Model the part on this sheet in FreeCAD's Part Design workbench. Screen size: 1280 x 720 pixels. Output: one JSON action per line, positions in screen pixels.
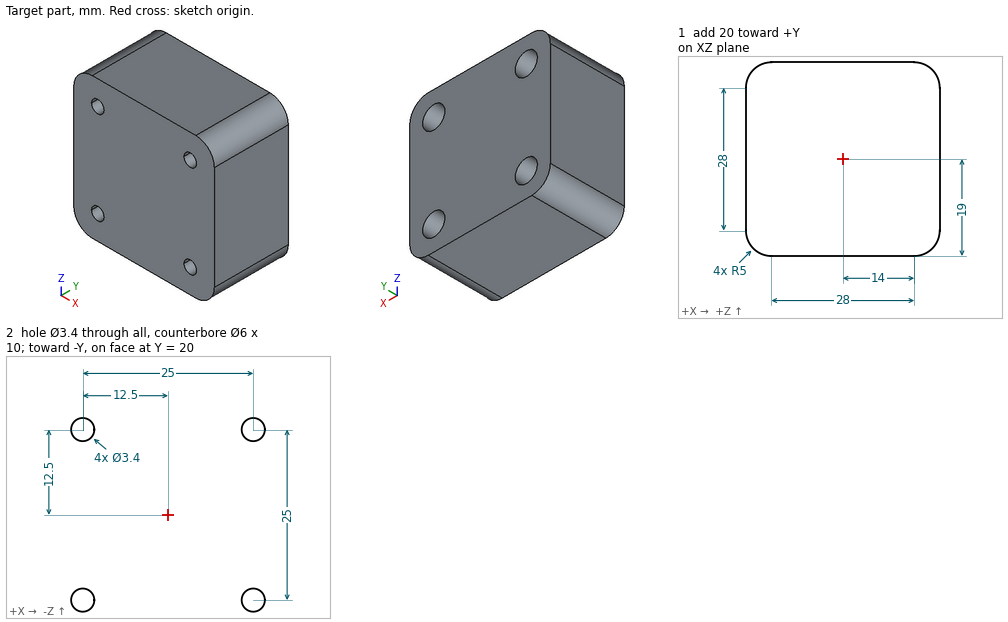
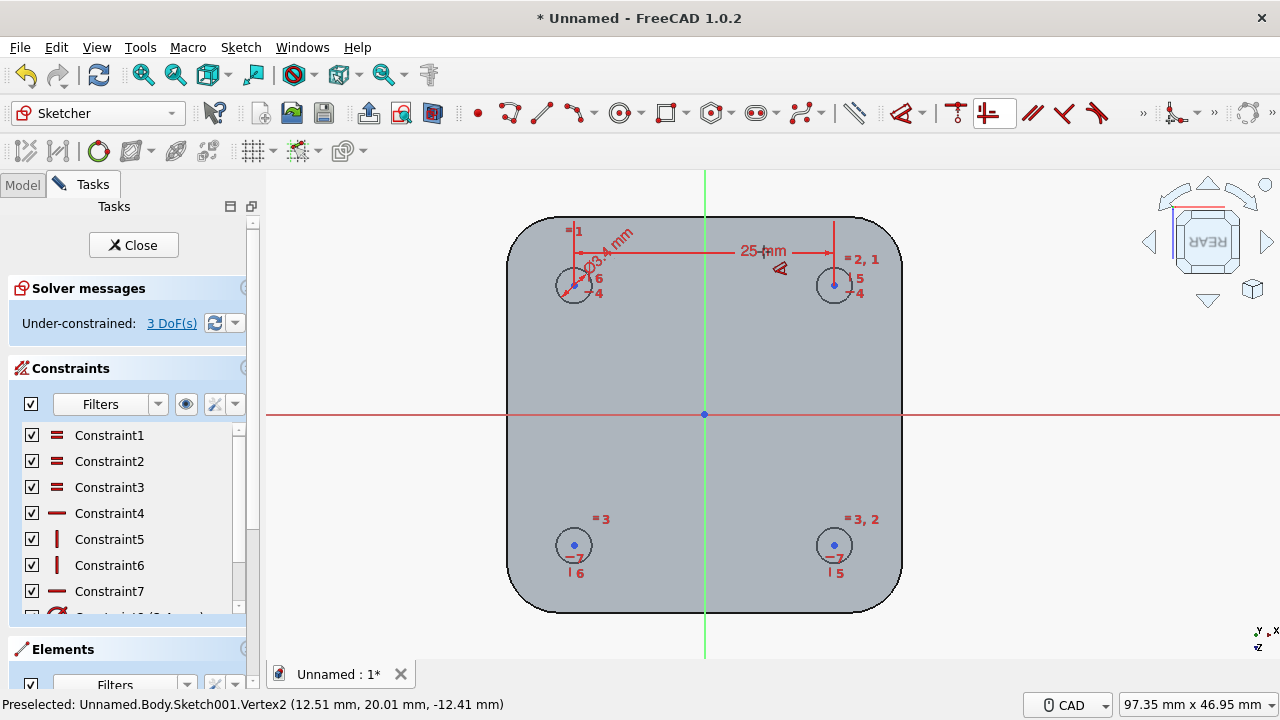
{"action": "left_click", "coordinate": [834, 286]}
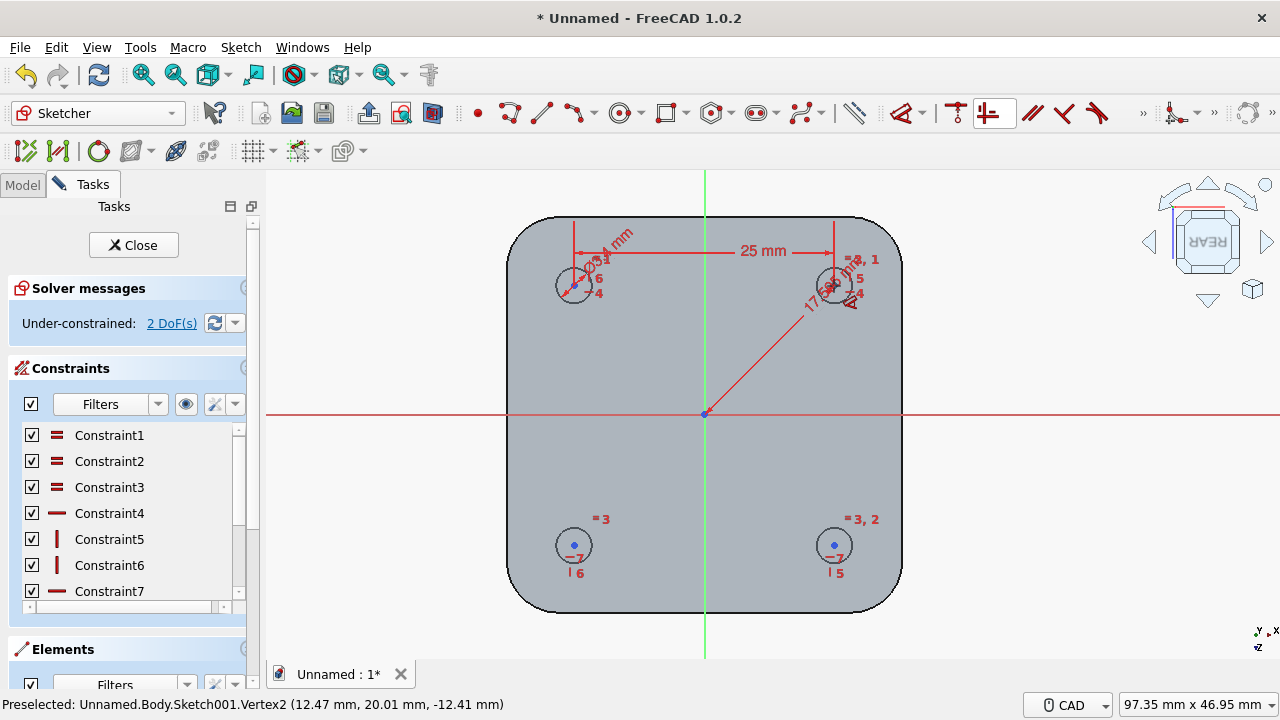
{"action": "left_click", "coordinate": [834, 546]}
{"action": "left_click", "coordinate": [868, 356]}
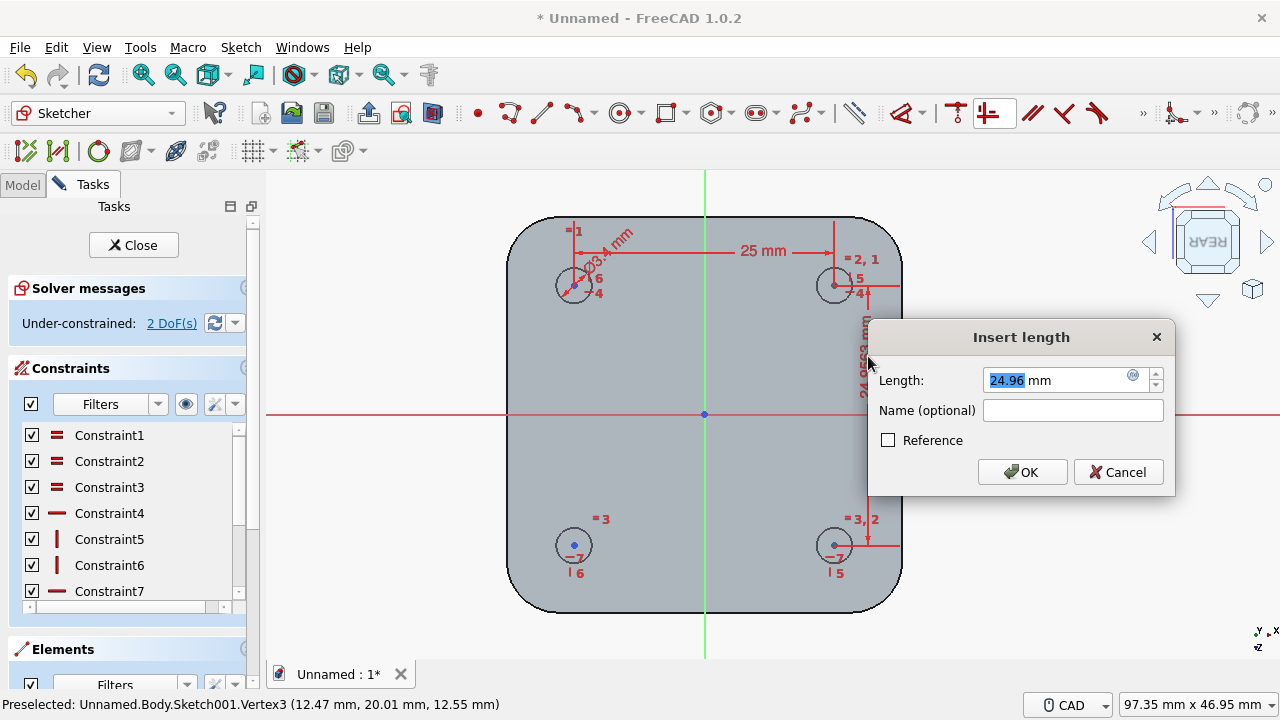
{"action": "type", "text": "25"}
{"action": "key", "text": "Return"}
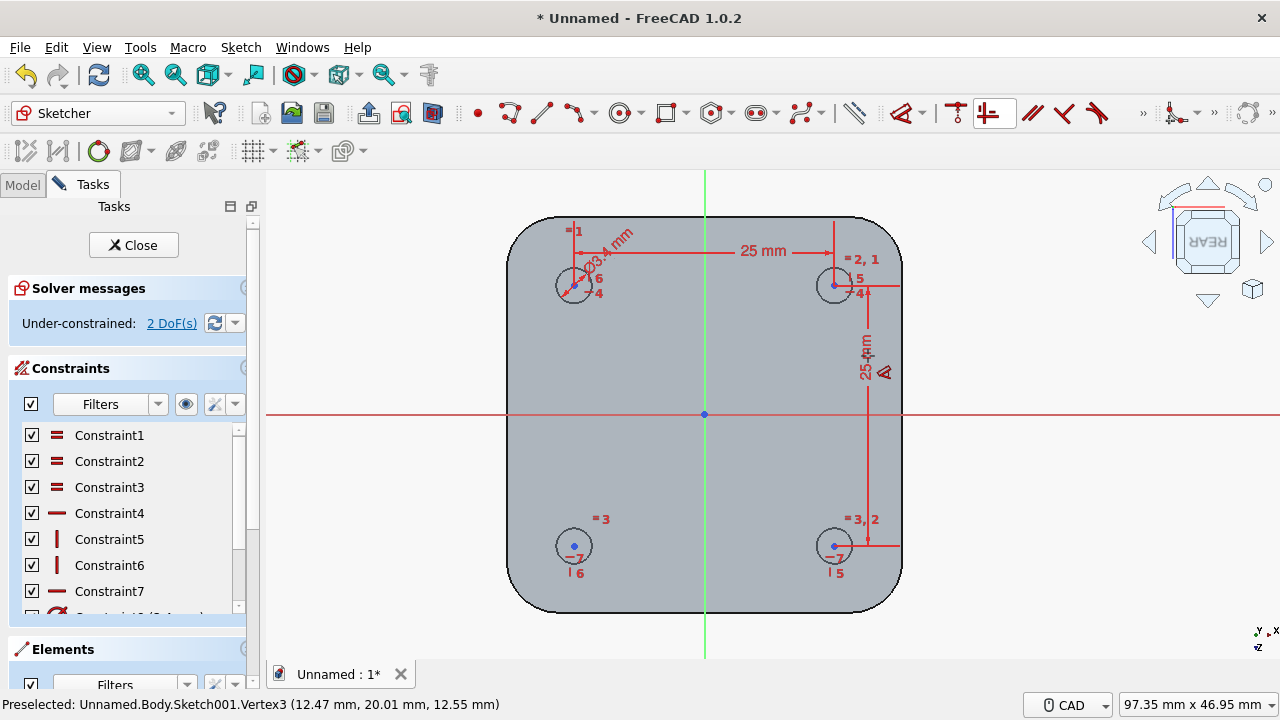
{"action": "left_click", "coordinate": [574, 286]}
{"action": "left_click", "coordinate": [685, 252]}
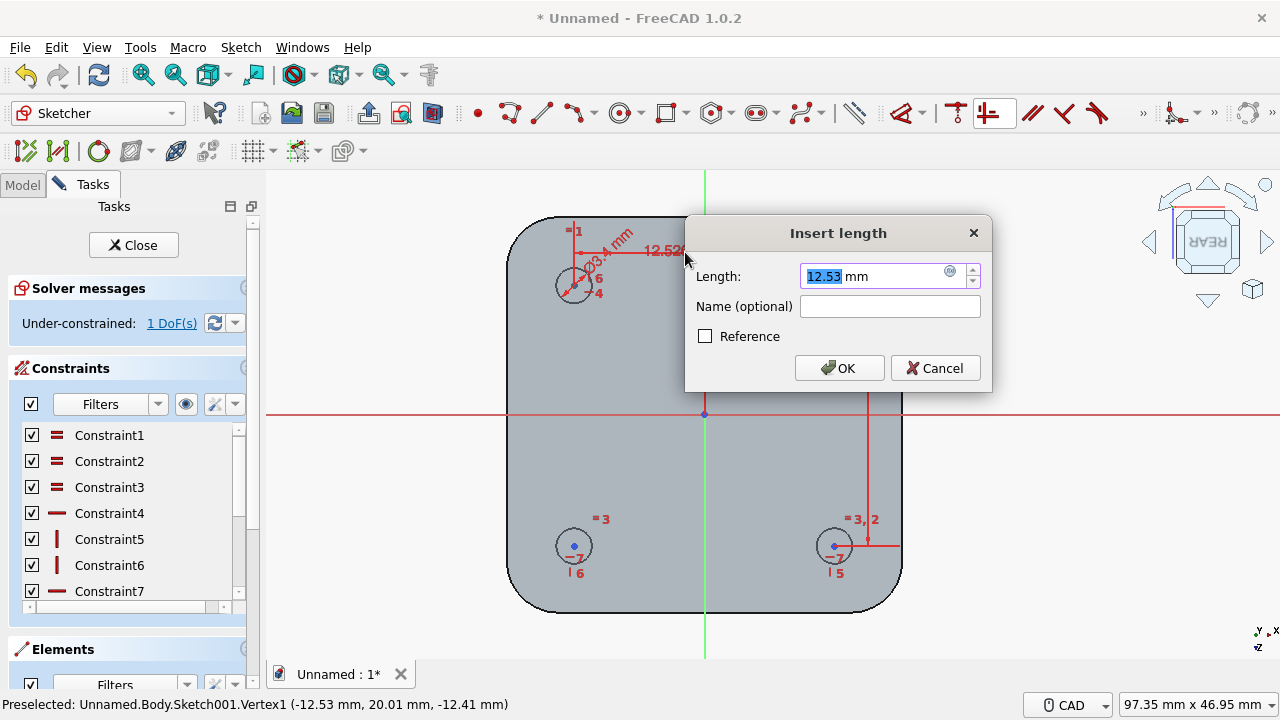
{"action": "type", "text": "12.5"}
{"action": "key", "text": "Return"}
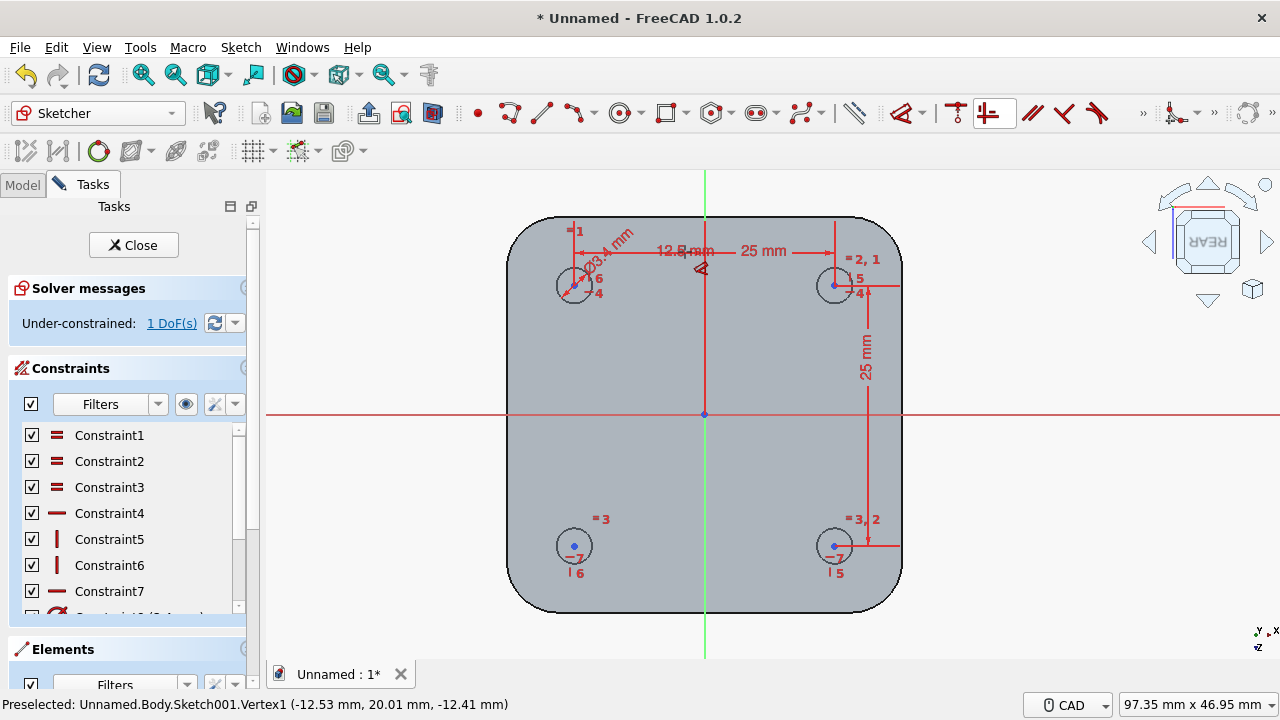
{"action": "left_click", "coordinate": [574, 286]}
{"action": "left_click", "coordinate": [540, 350]}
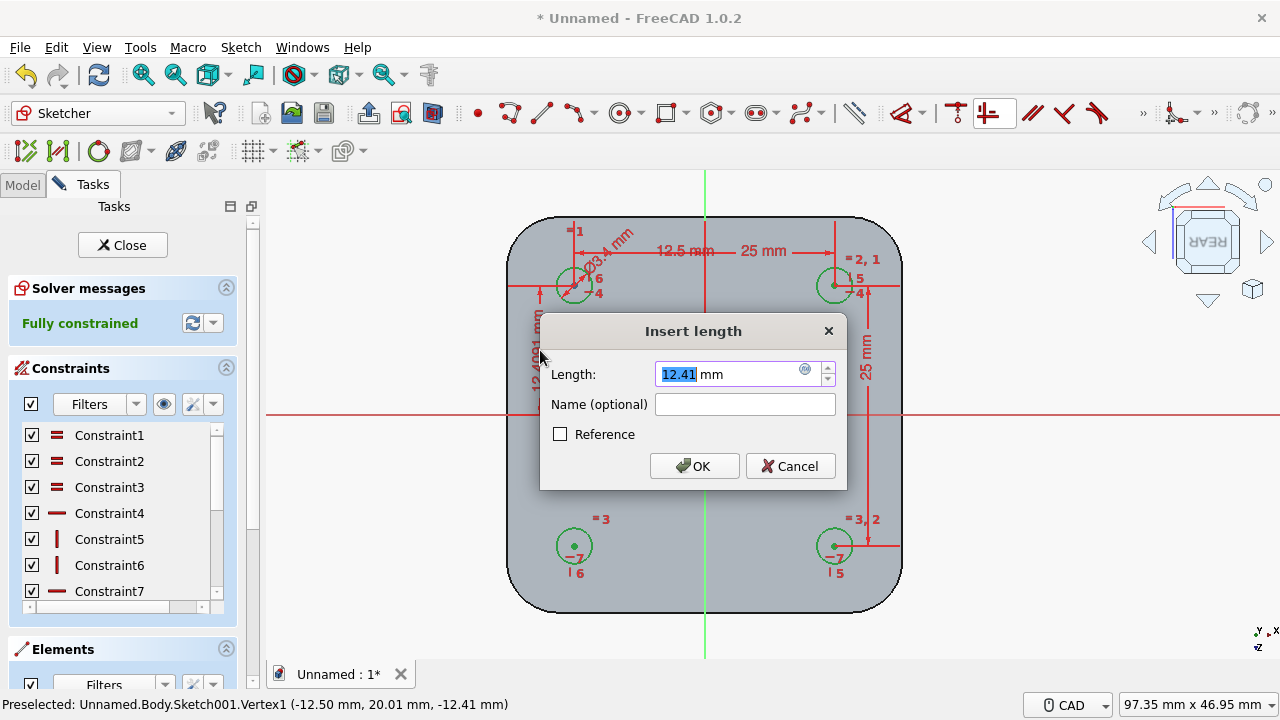
{"action": "type", "text": "12.5"}
{"action": "key", "text": "Return"}
{"action": "key", "text": "Escape"}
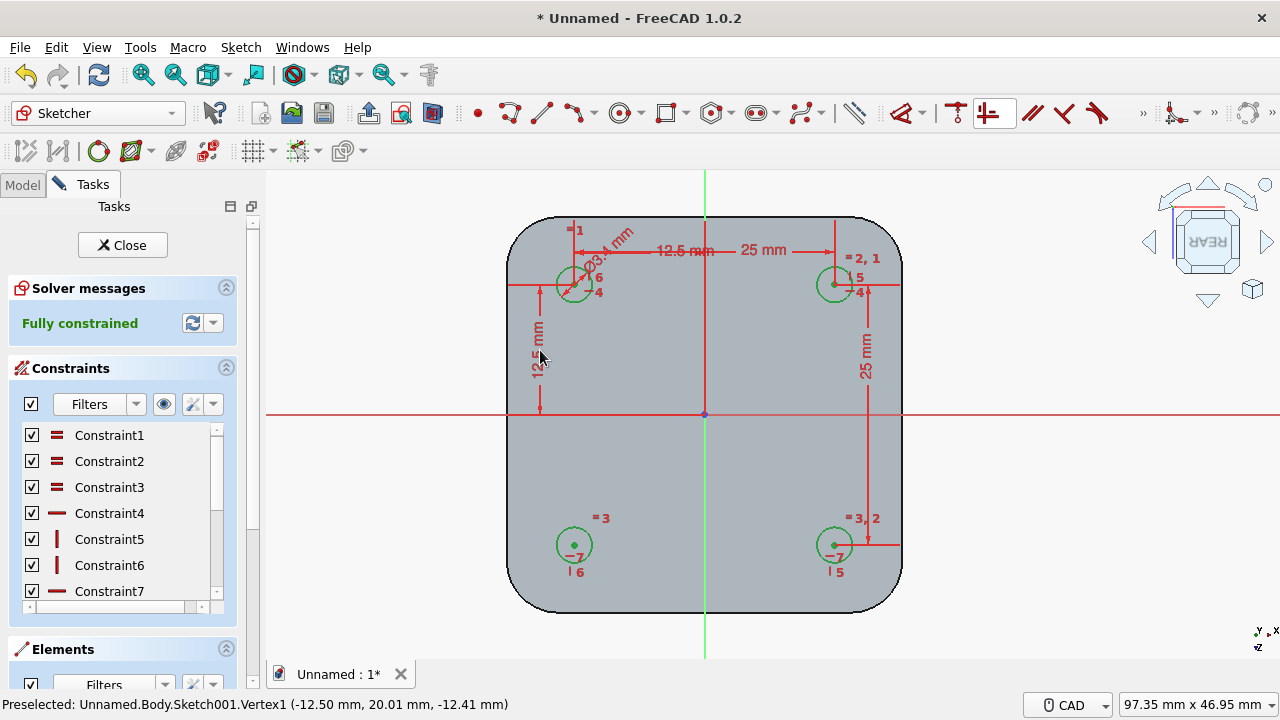
{"action": "left_click", "coordinate": [123, 245]}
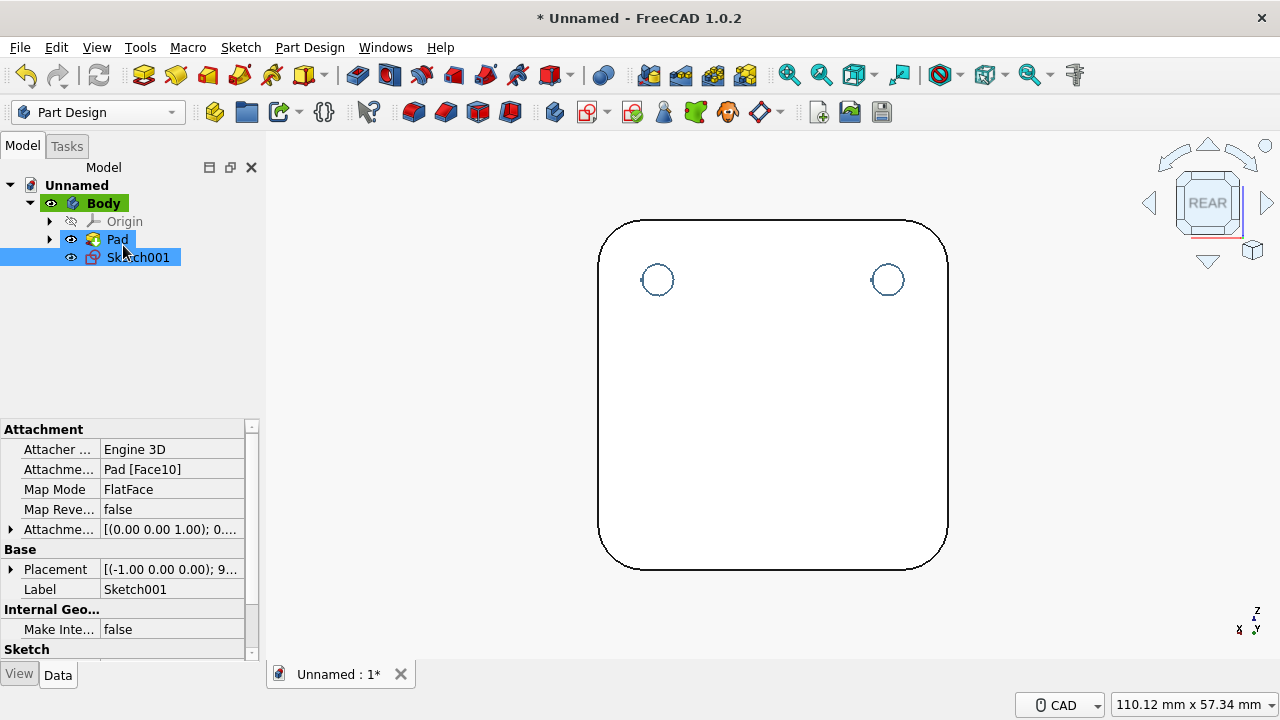
{"action": "left_click", "coordinate": [390, 76]}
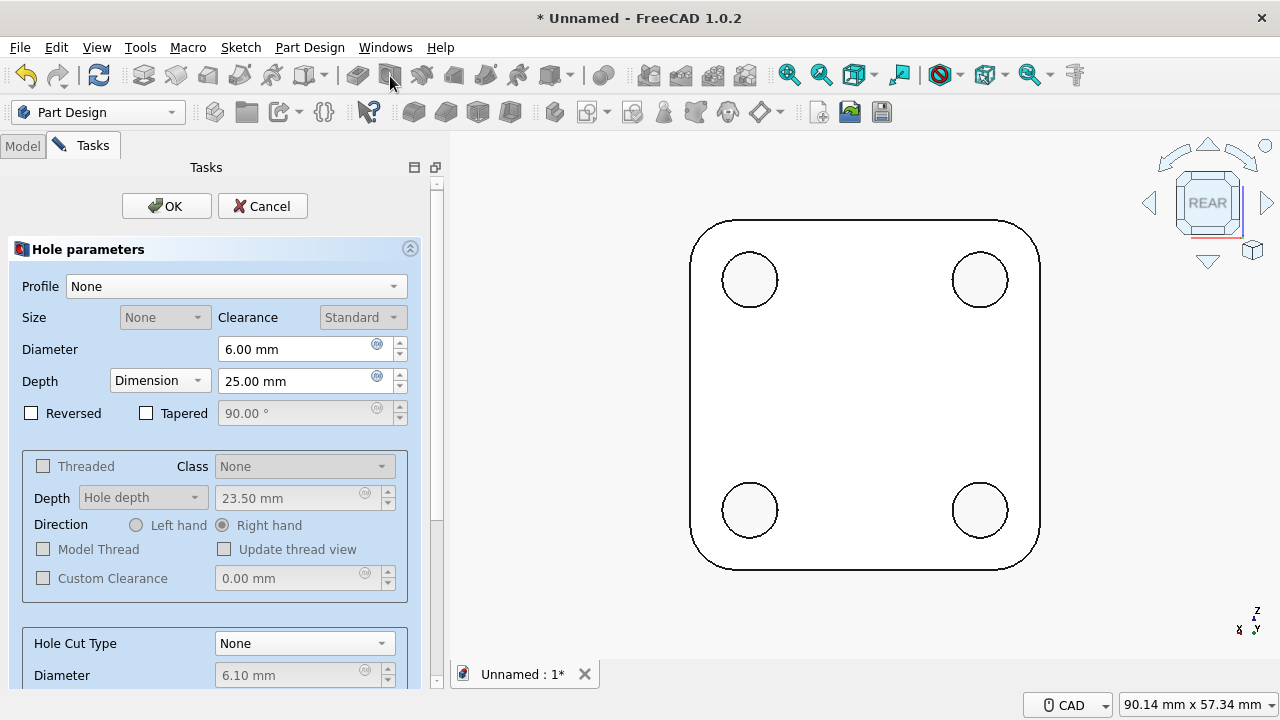
{"action": "triple_click", "coordinate": [305, 349]}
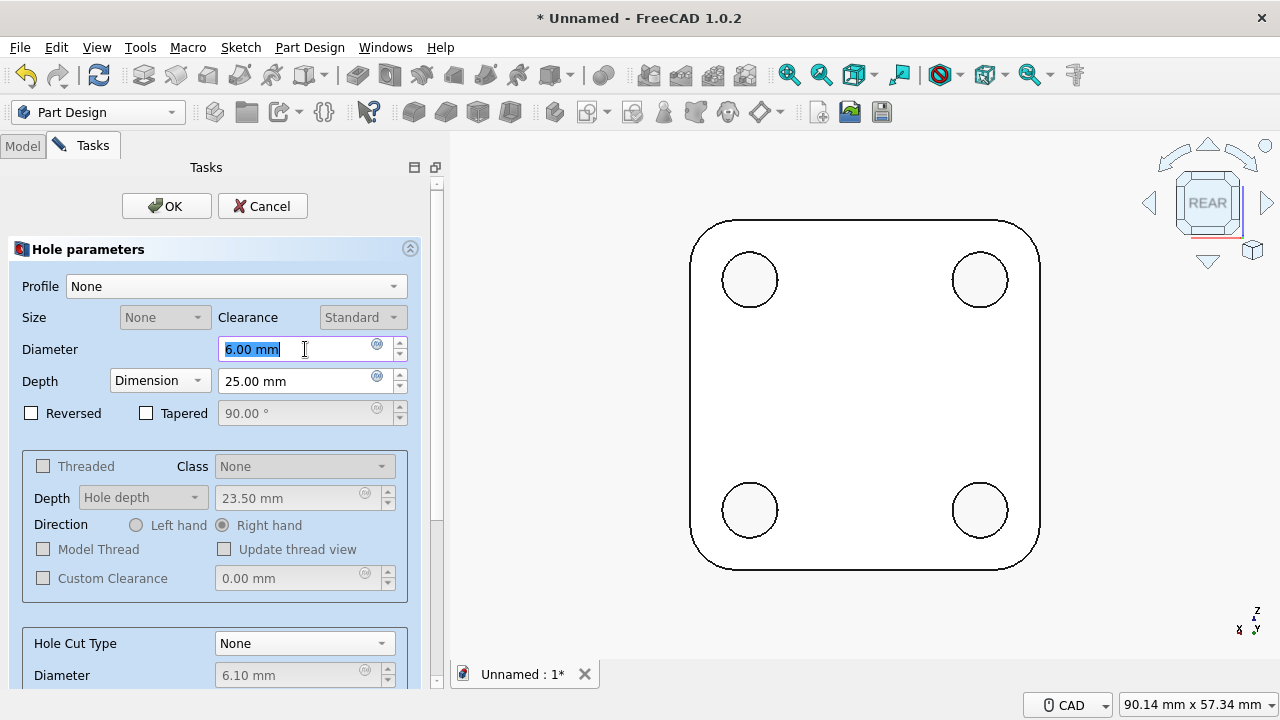
{"action": "type", "text": "3.4"}
{"action": "key", "text": "Tab"}